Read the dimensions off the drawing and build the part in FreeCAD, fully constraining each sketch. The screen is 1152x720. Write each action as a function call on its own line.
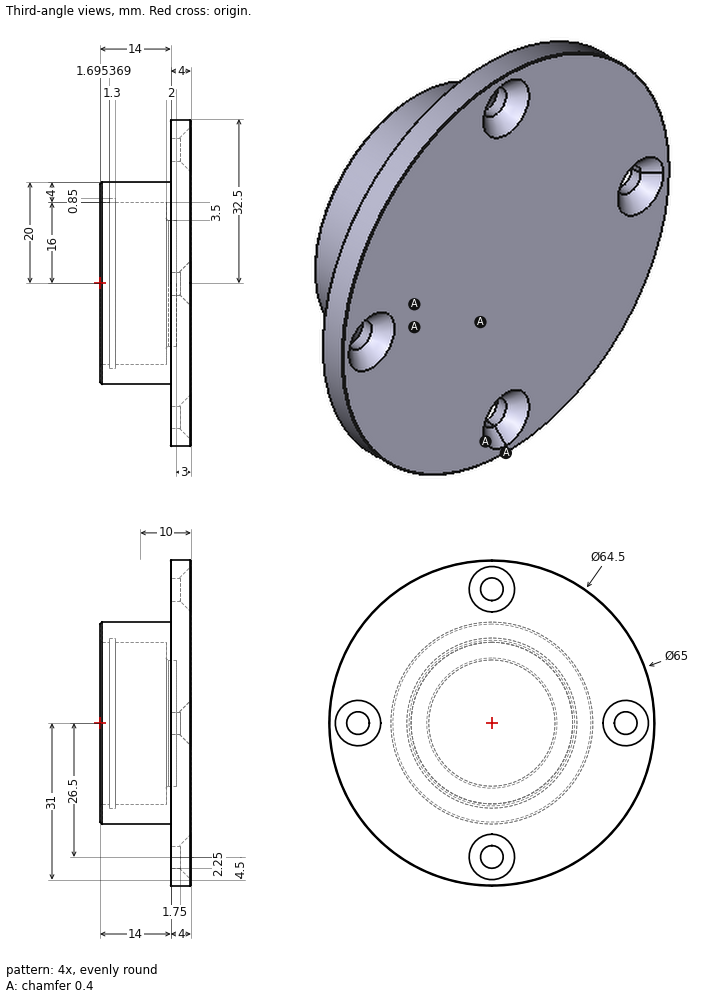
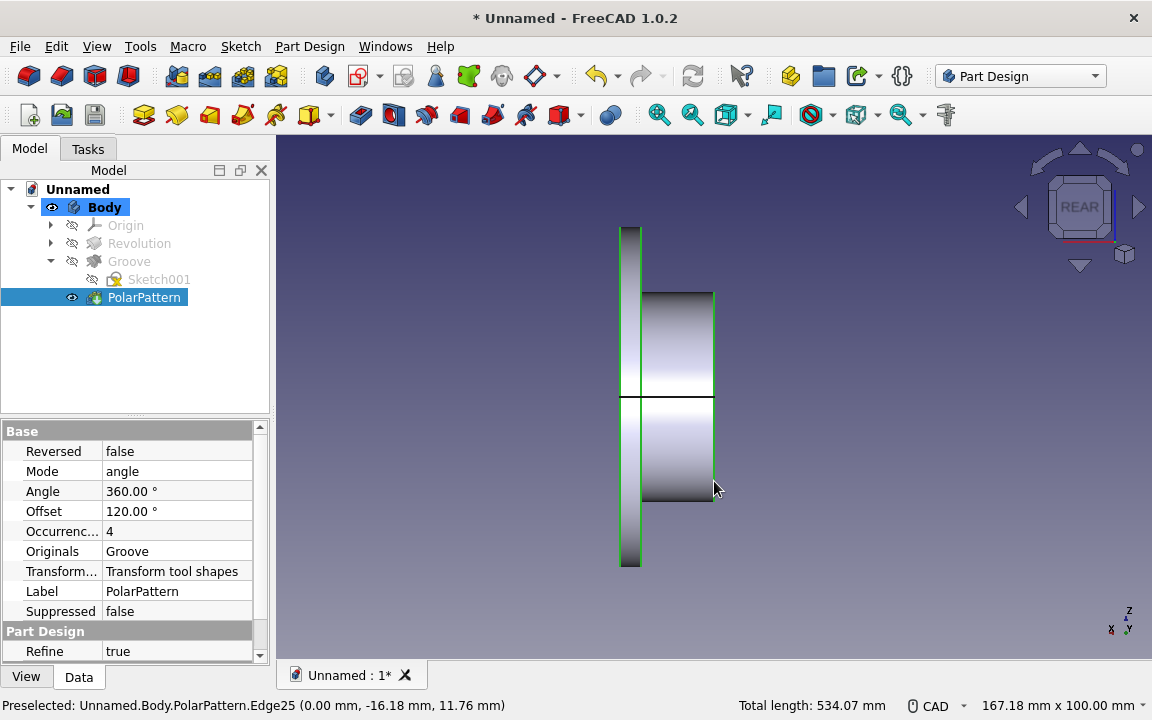
key(6)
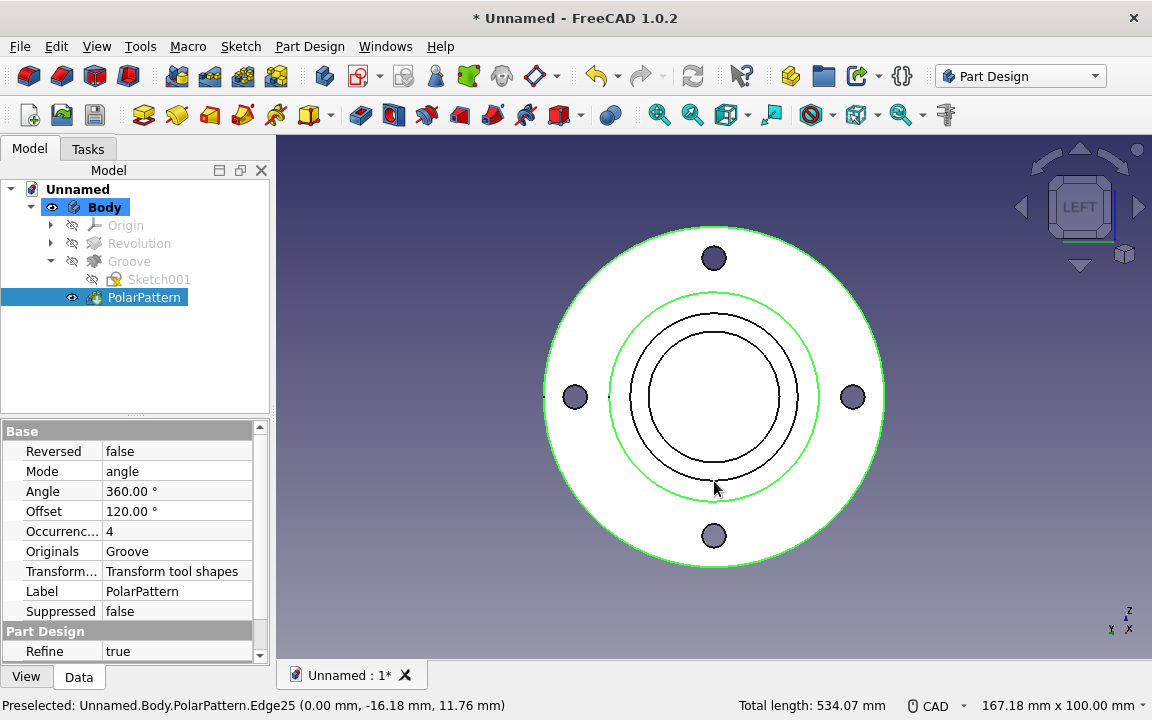
click(780, 396, ctrl)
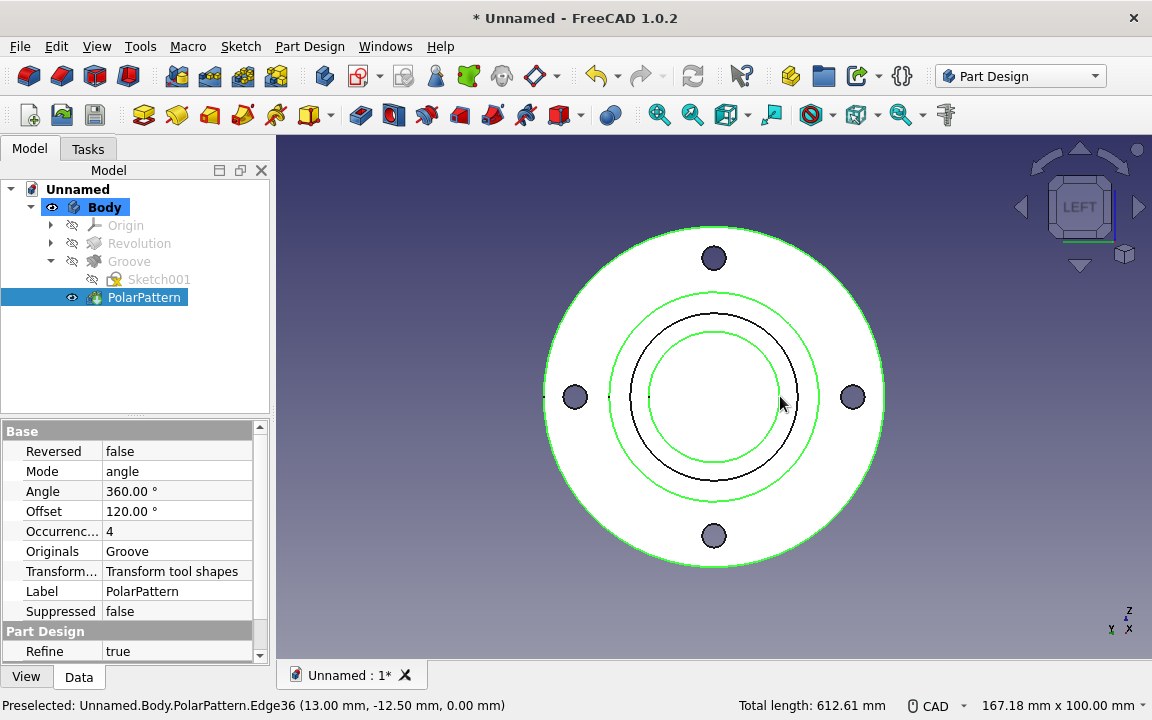
click(782, 445, ctrl)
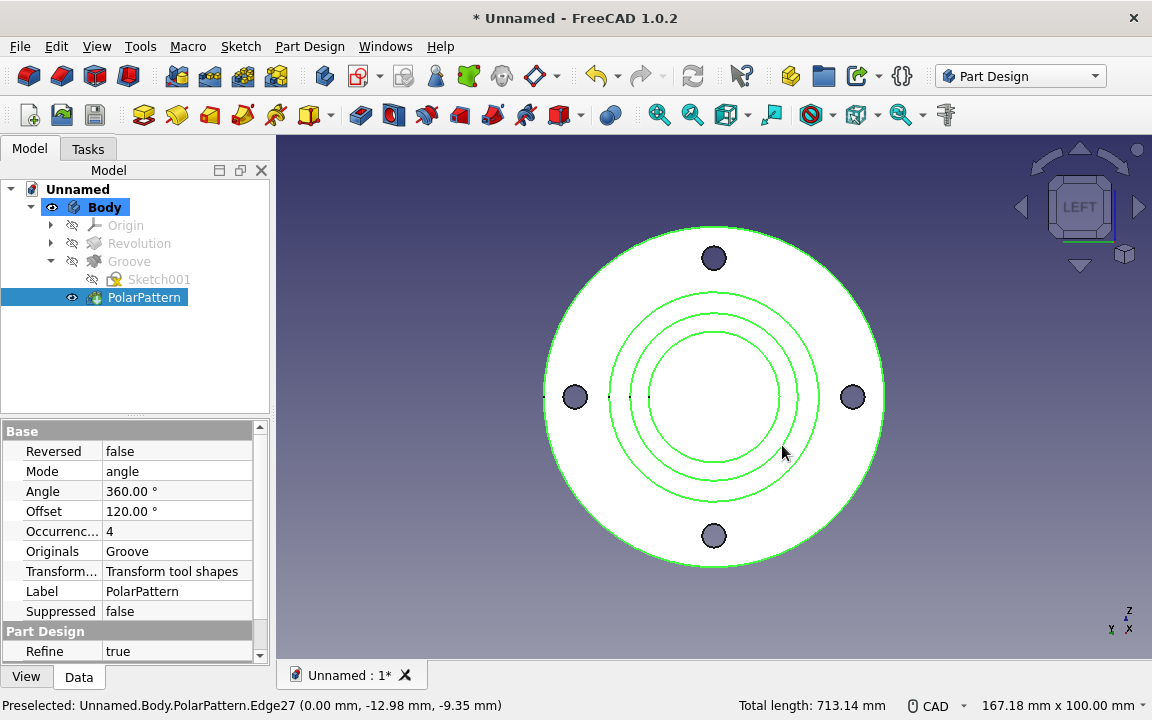
click(62, 76)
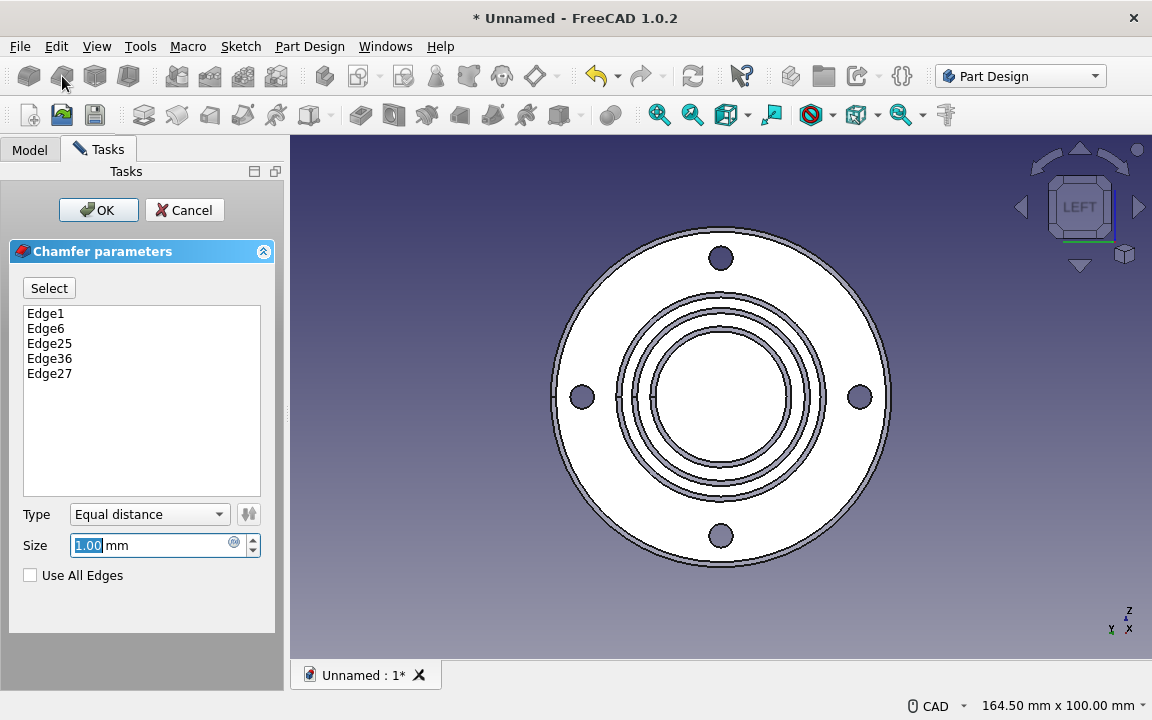
text(0.4)
key(Tab)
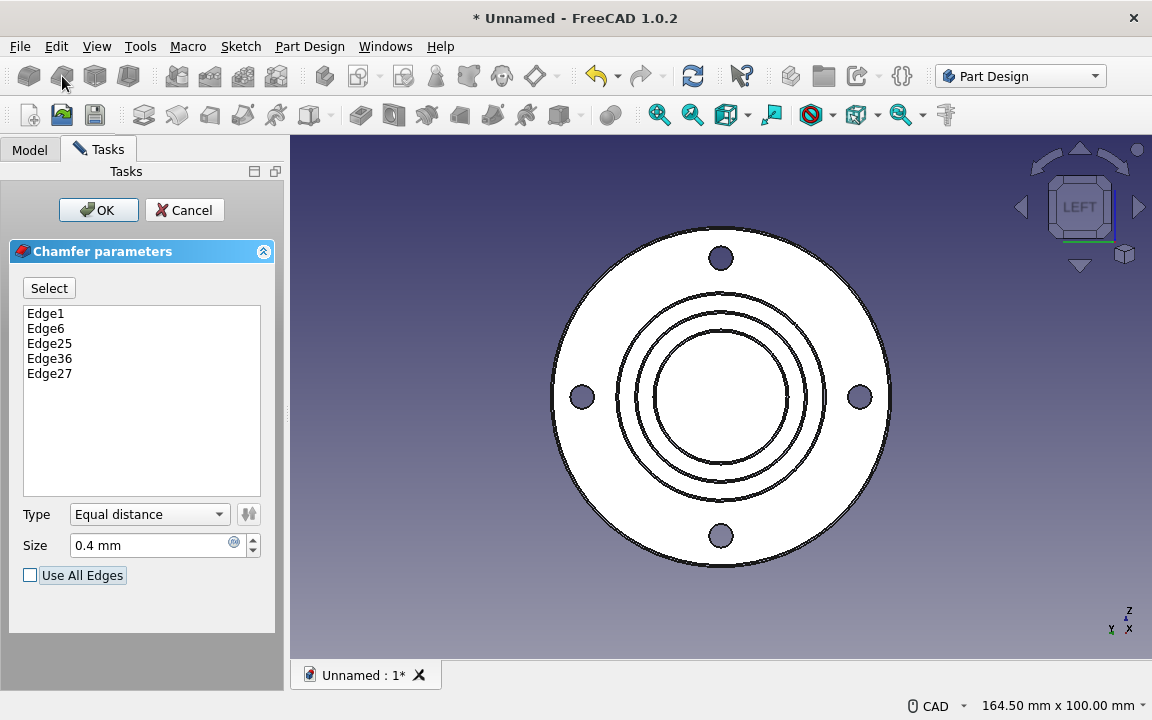
click(99, 210)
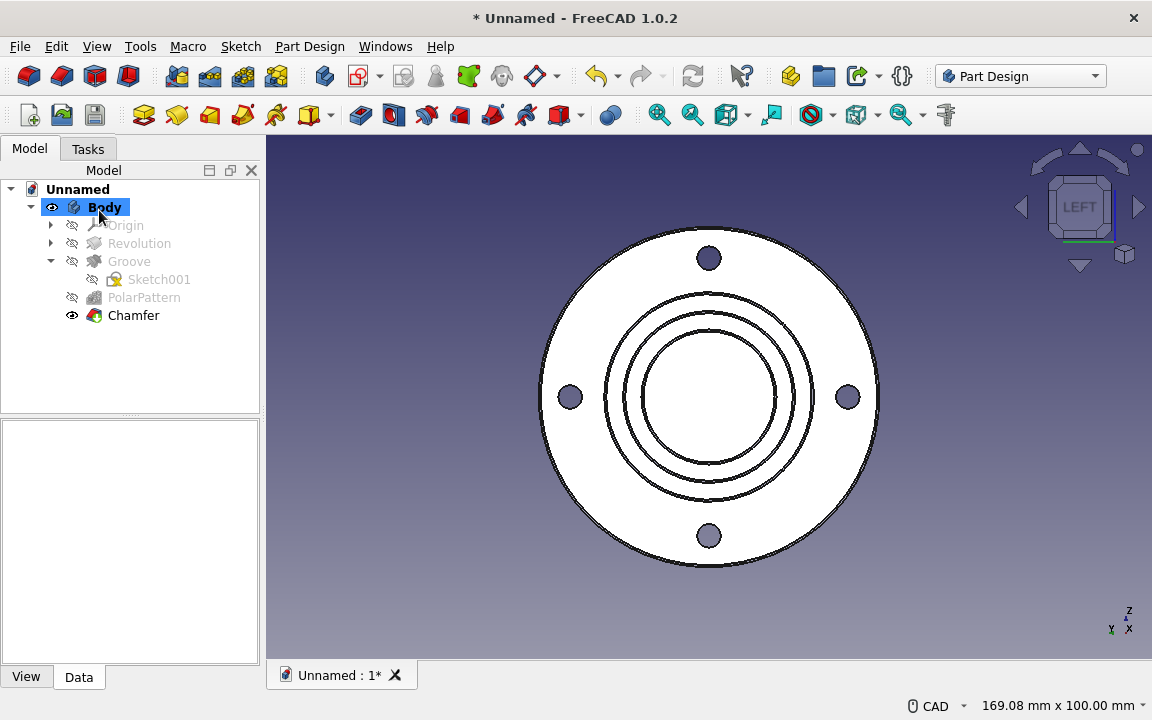
click(51, 225)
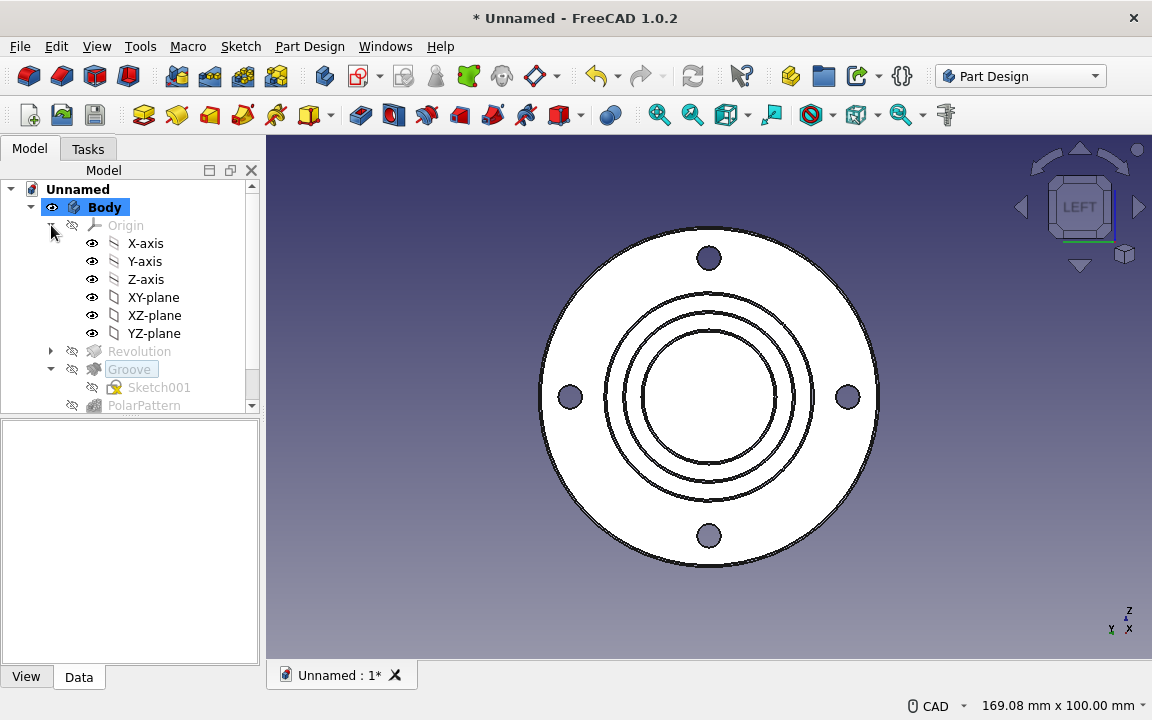
click(137, 333)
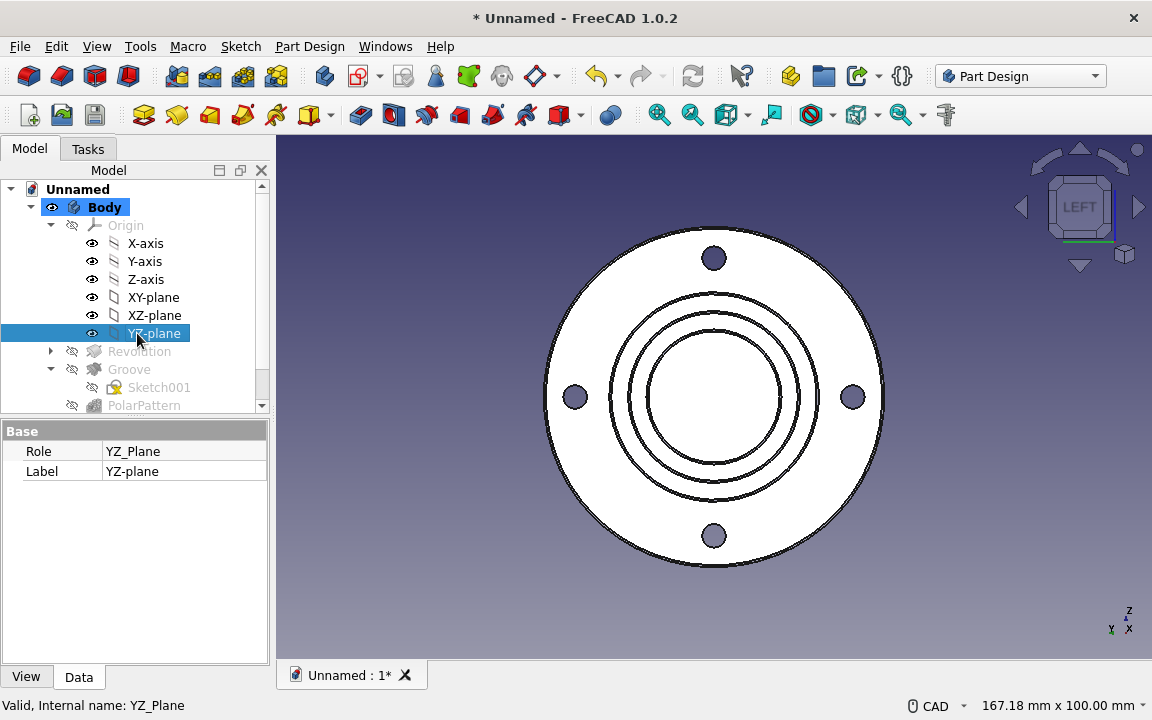
click(534, 76)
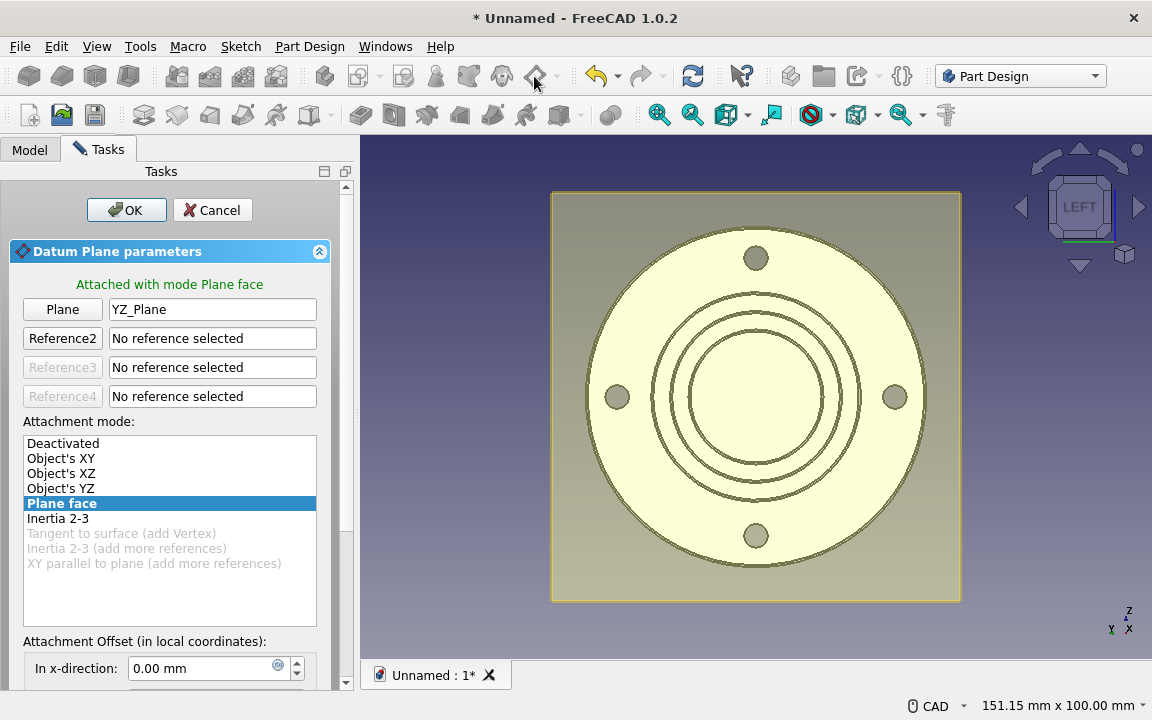
scroll(346, 436, down, 2)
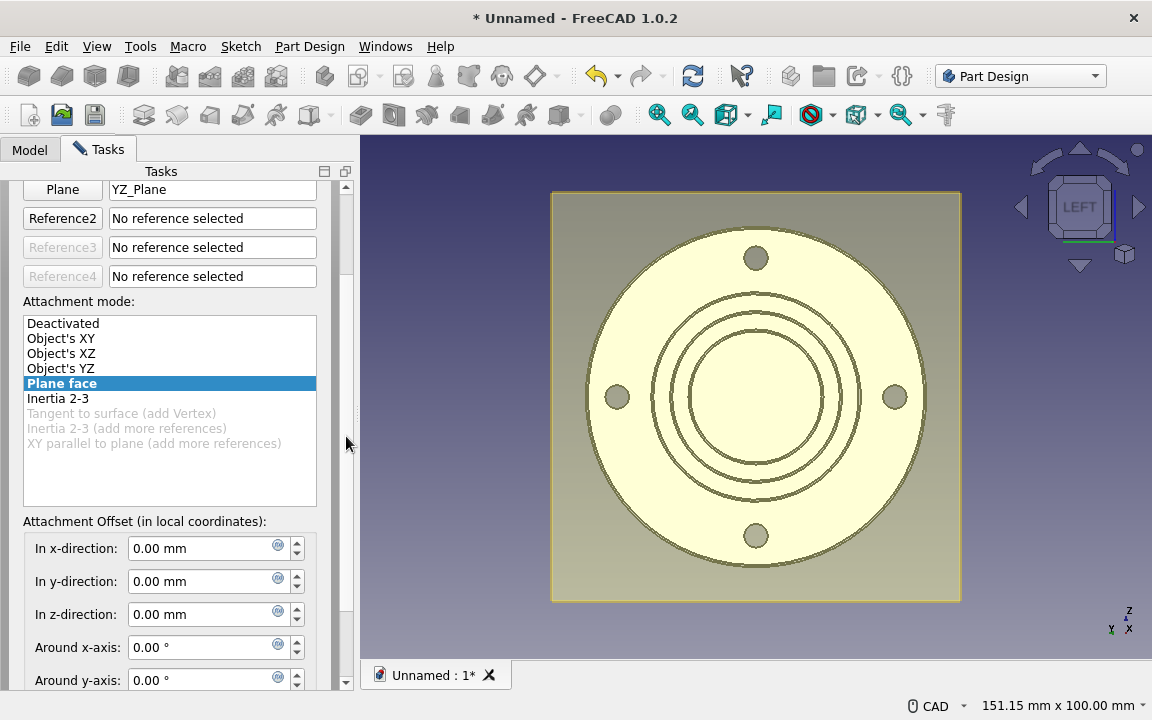
triple_click(210, 614)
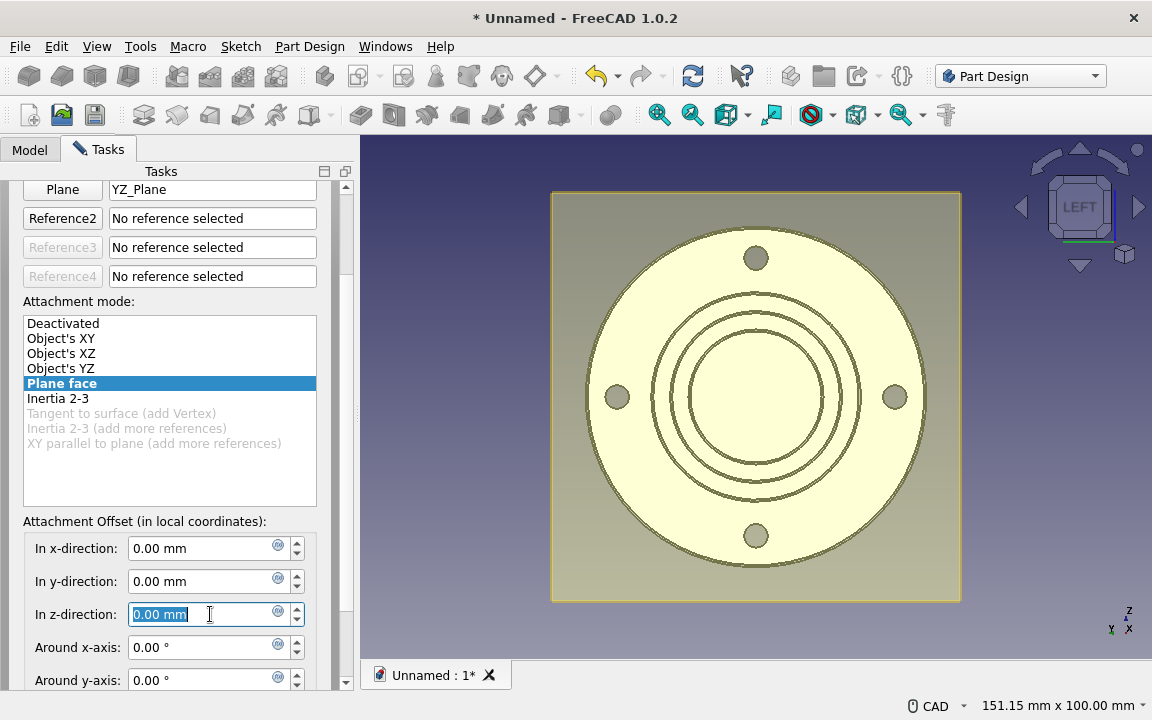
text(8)
key(Tab)